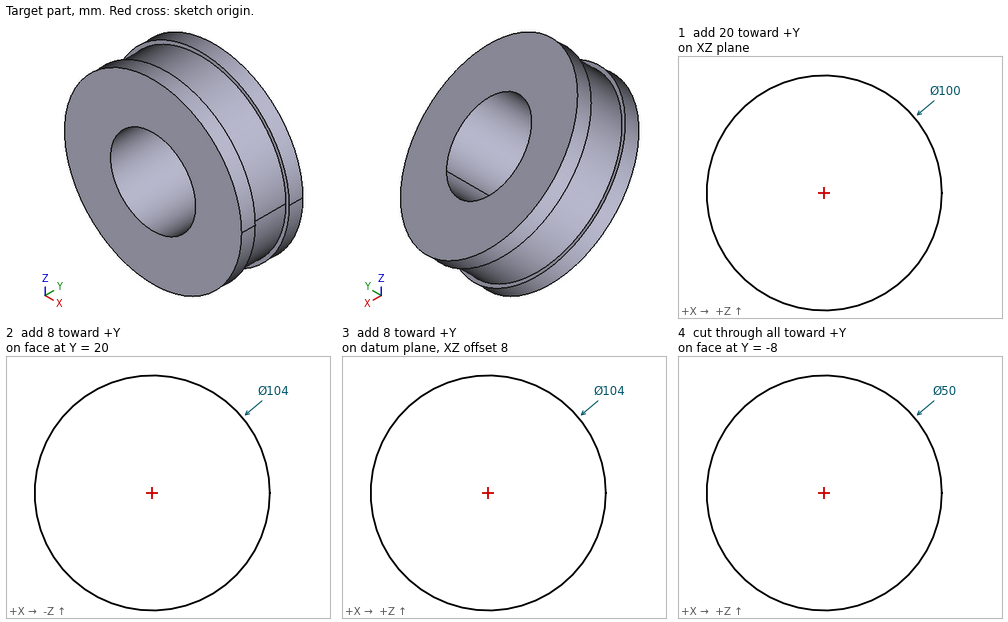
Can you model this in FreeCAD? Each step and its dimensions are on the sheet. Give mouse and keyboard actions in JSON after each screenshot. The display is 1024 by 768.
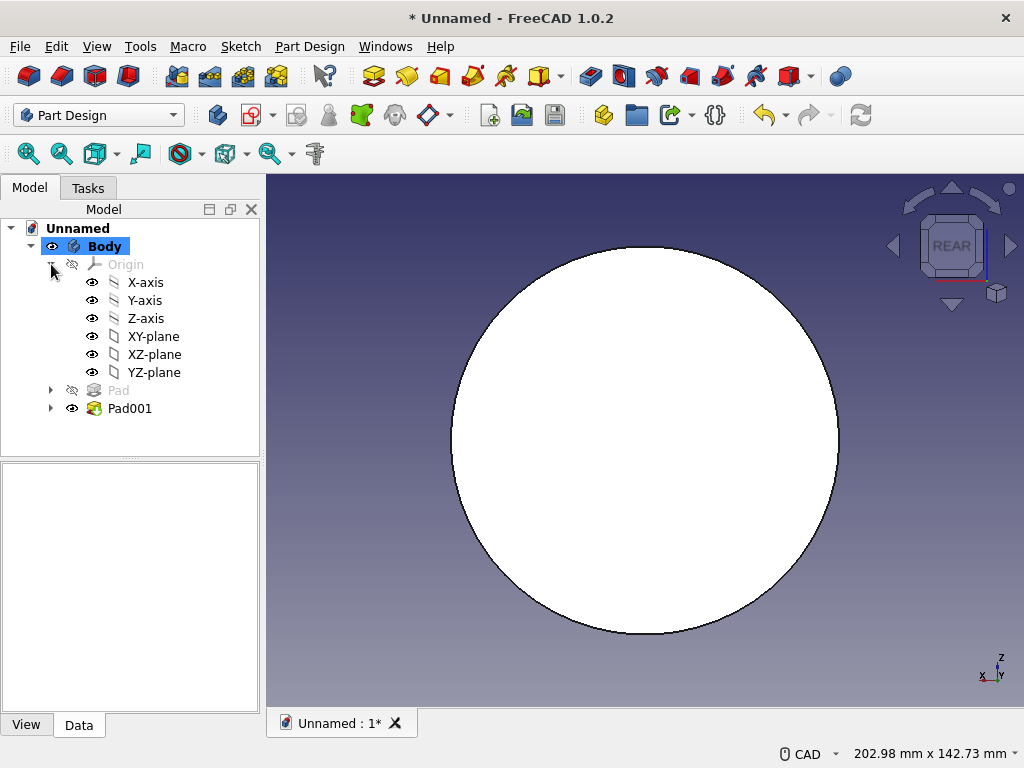
{"action": "left_click", "coordinate": [137, 354]}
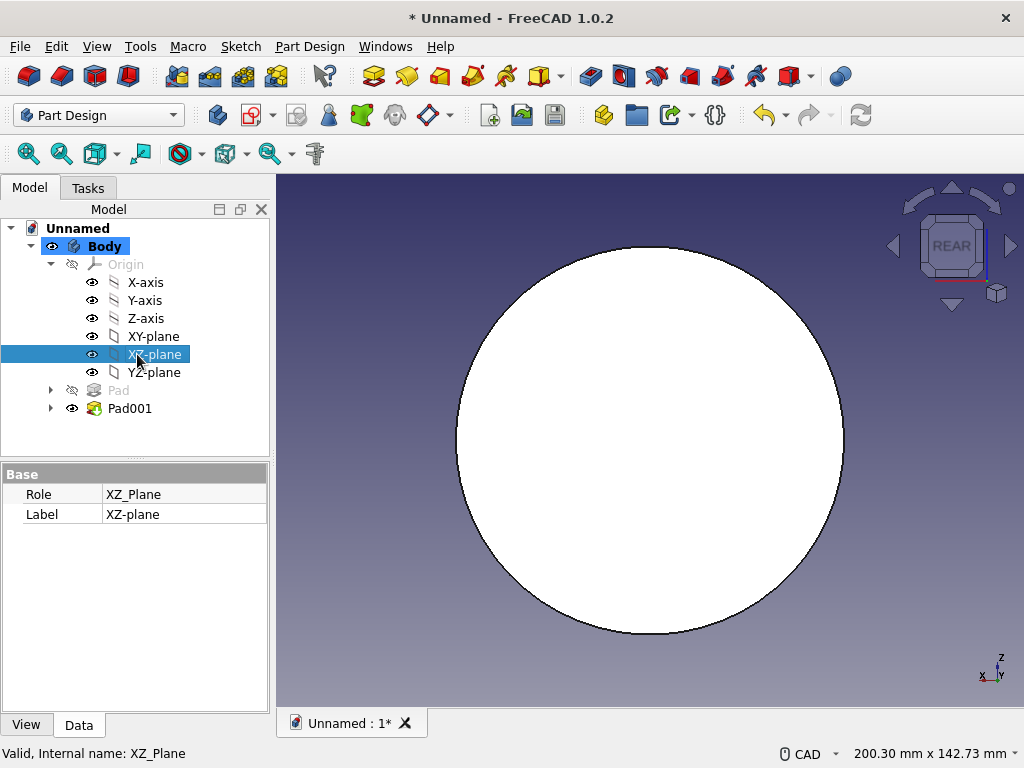
{"action": "left_click", "coordinate": [428, 116]}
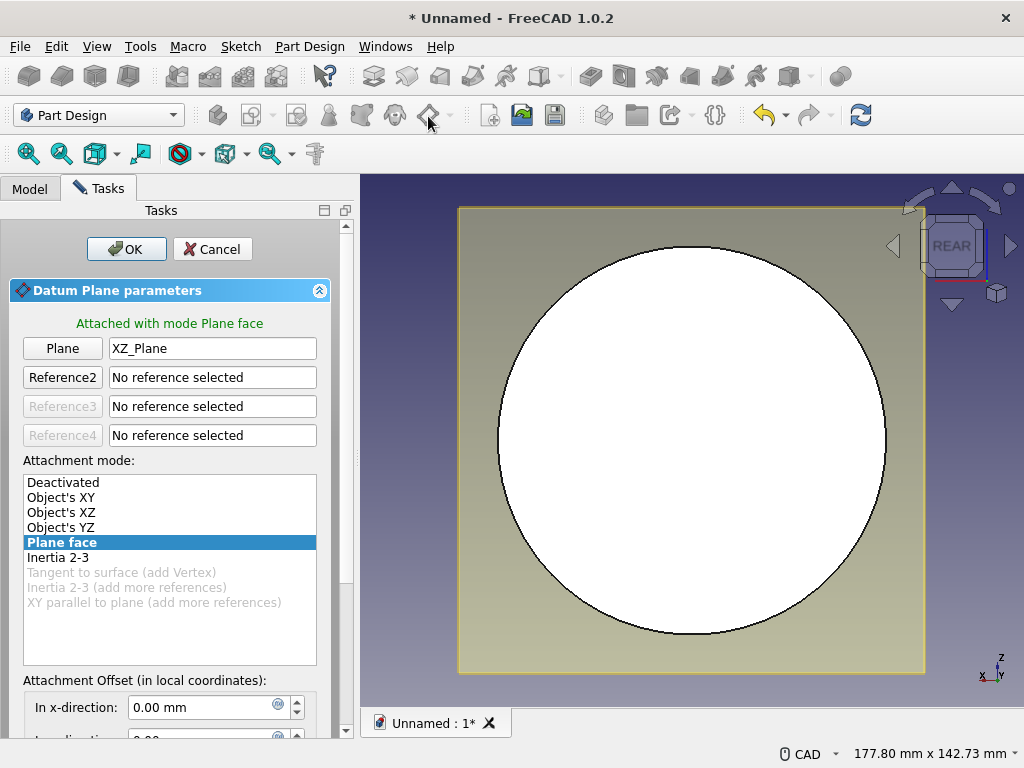
{"action": "scroll", "coordinate": [346, 479], "scroll_direction": "down", "scroll_amount": 2}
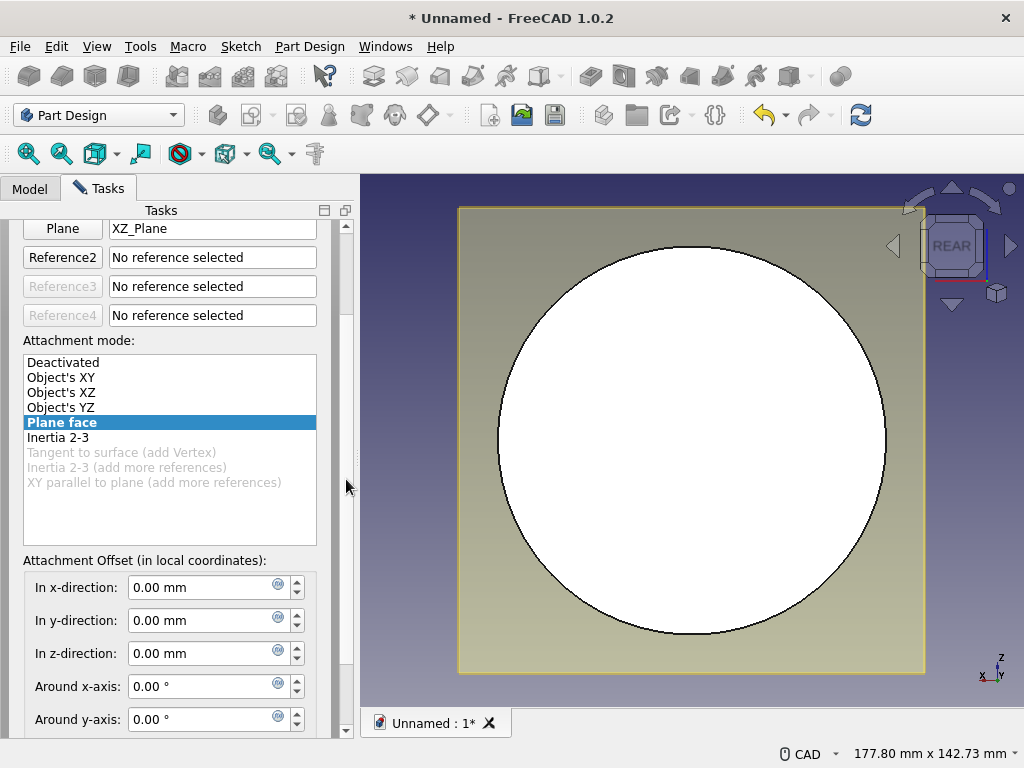
{"action": "triple_click", "coordinate": [210, 654]}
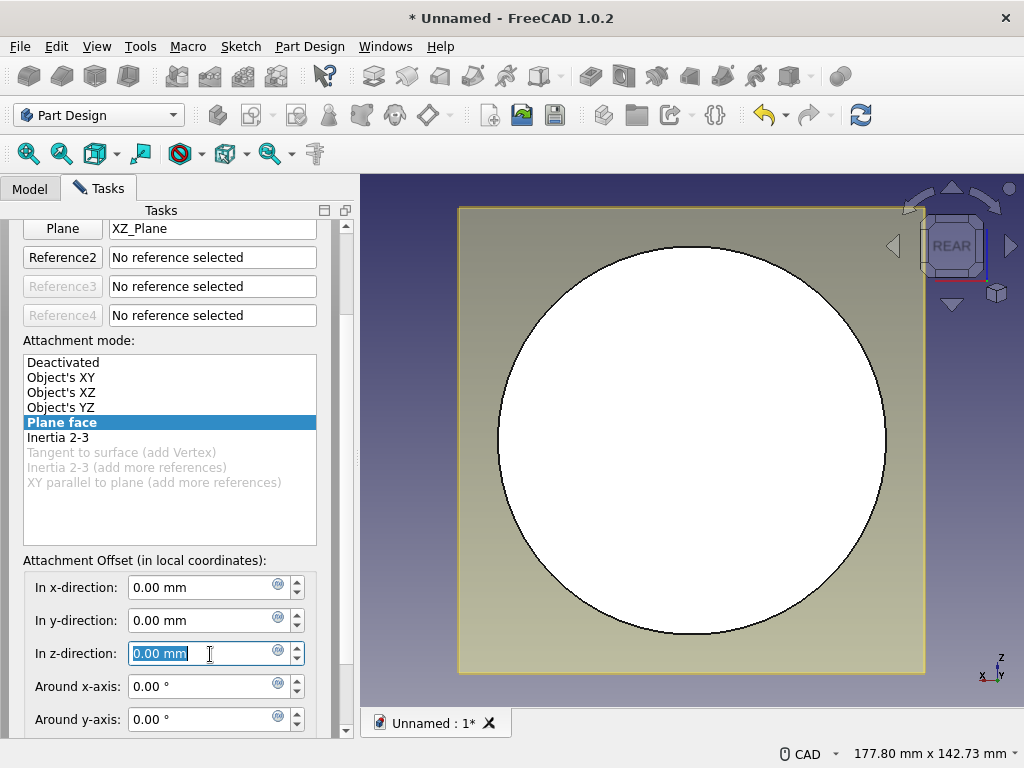
{"action": "type", "text": "8"}
{"action": "key", "text": "Tab"}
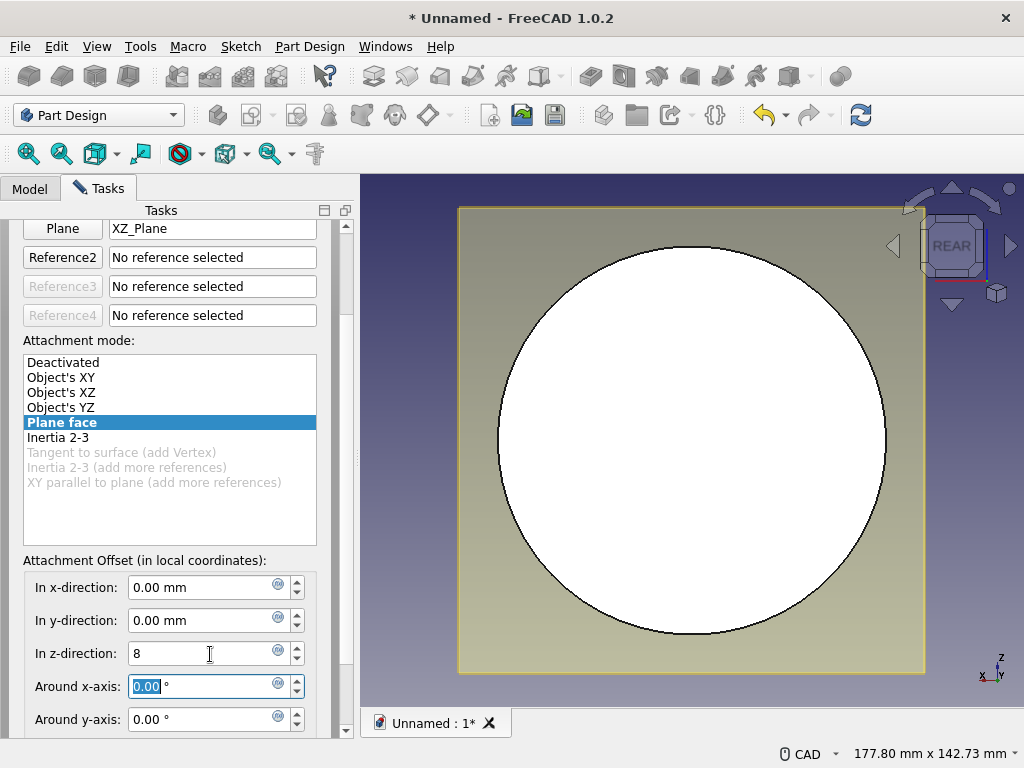
{"action": "scroll", "coordinate": [346, 479], "scroll_direction": "up", "scroll_amount": 3}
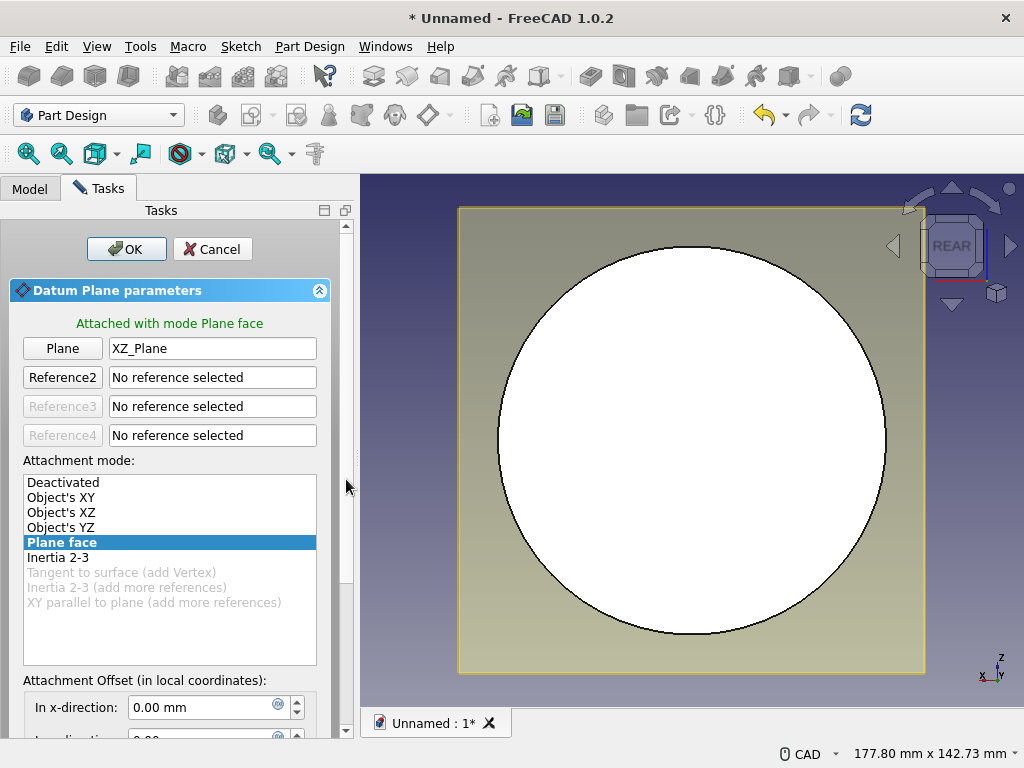
{"action": "left_click", "coordinate": [127, 249]}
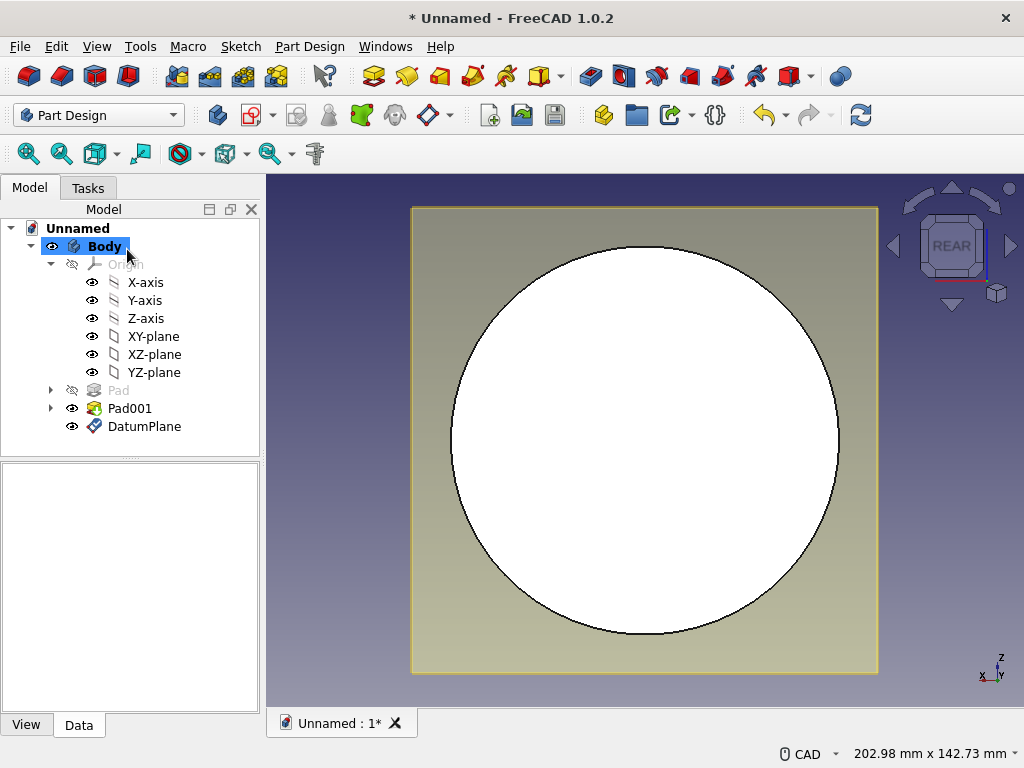
{"action": "left_click", "coordinate": [117, 426]}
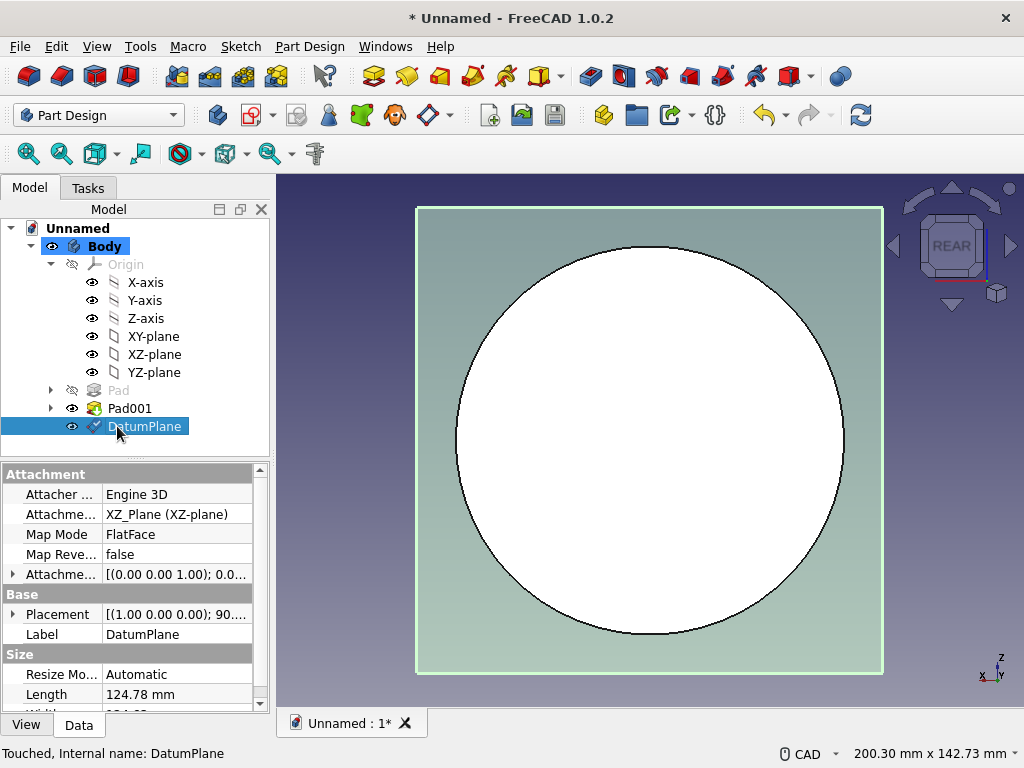
{"action": "left_click", "coordinate": [250, 116]}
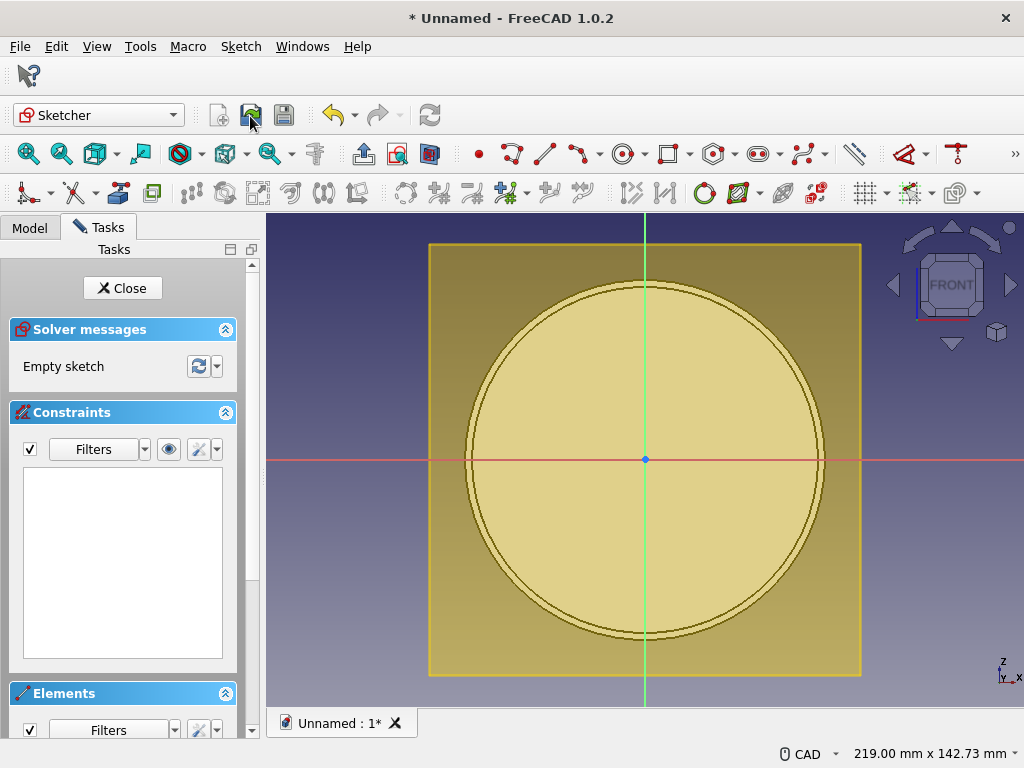
{"action": "left_click", "coordinate": [622, 154]}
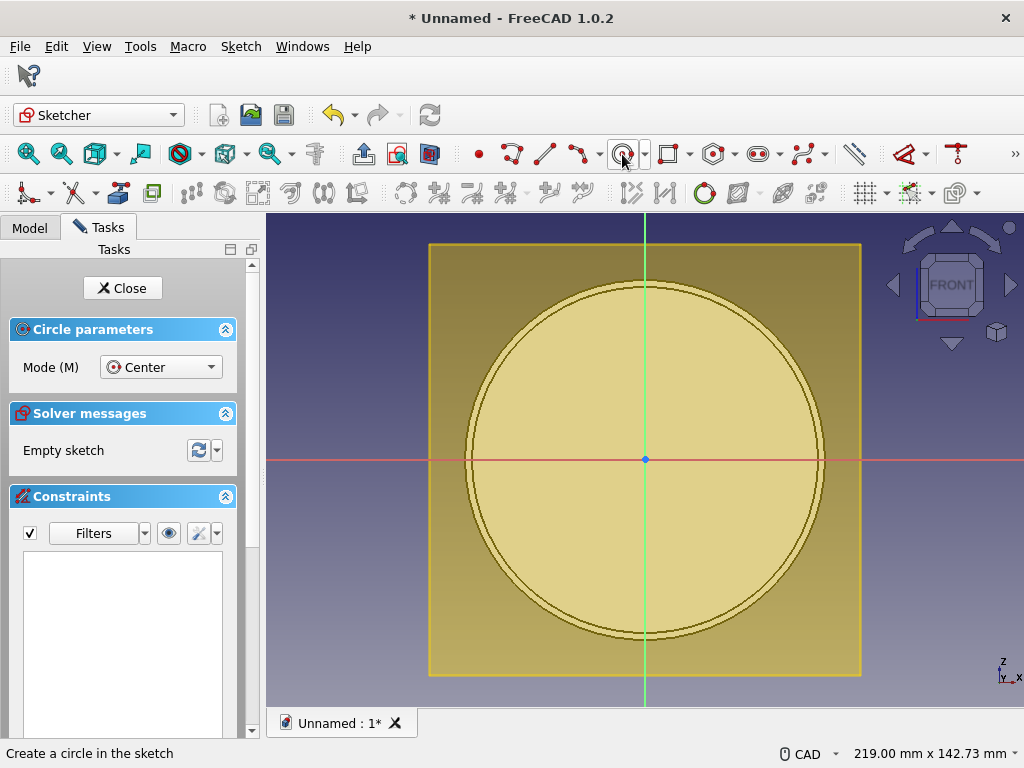
{"action": "left_click", "coordinate": [645, 460]}
{"action": "mouse_move", "coordinate": [772, 333]}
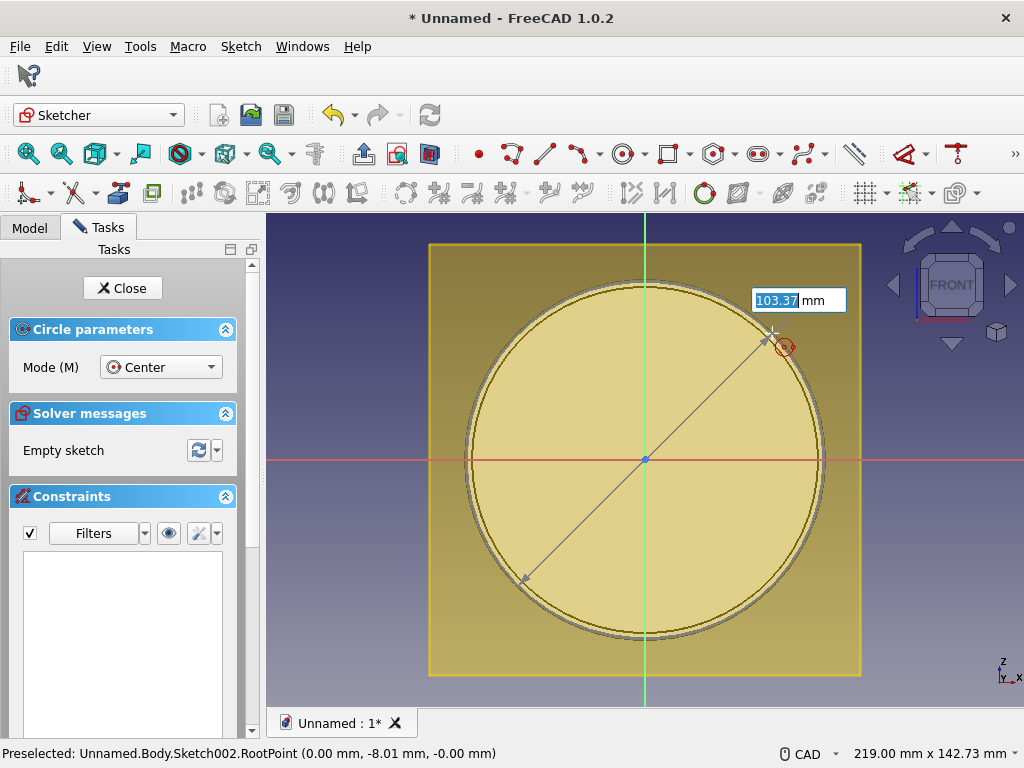
{"action": "type", "text": "104"}
{"action": "key", "text": "Return"}
{"action": "key", "text": "Escape"}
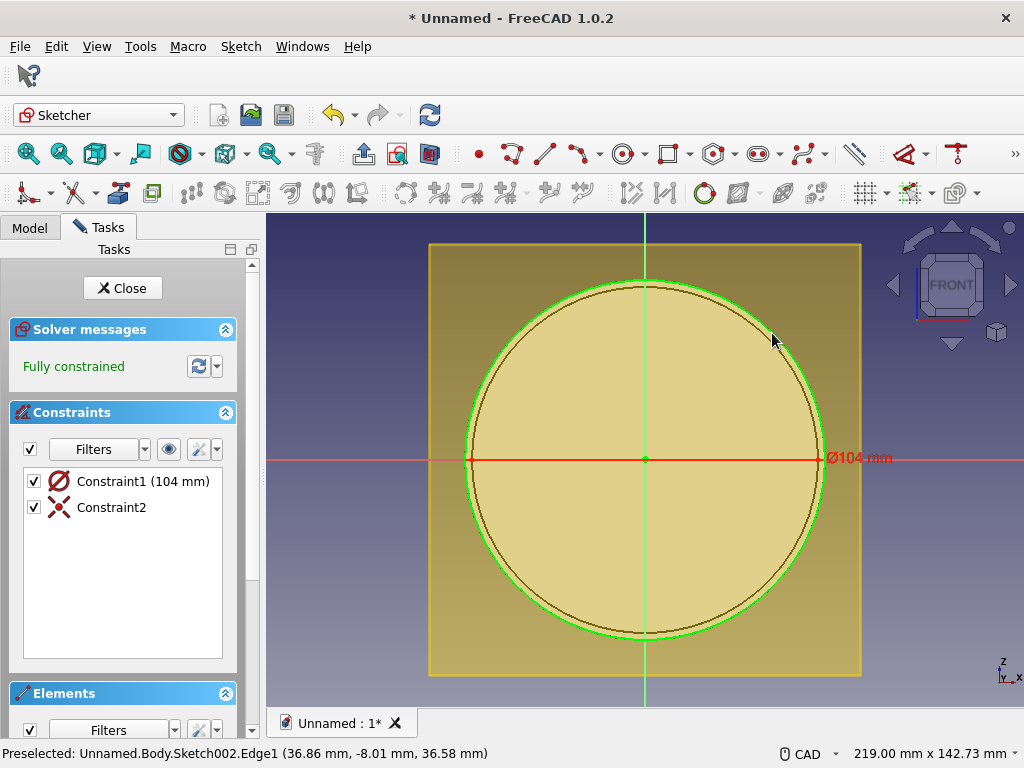
{"action": "left_click", "coordinate": [123, 288]}